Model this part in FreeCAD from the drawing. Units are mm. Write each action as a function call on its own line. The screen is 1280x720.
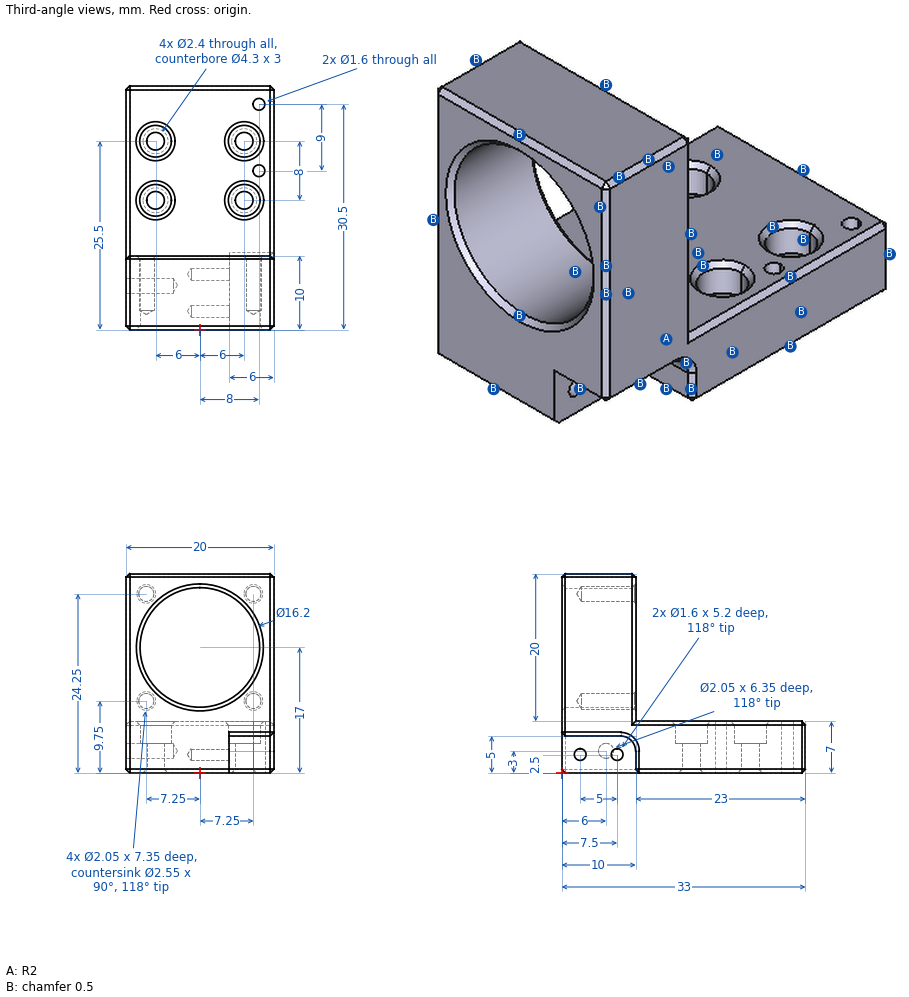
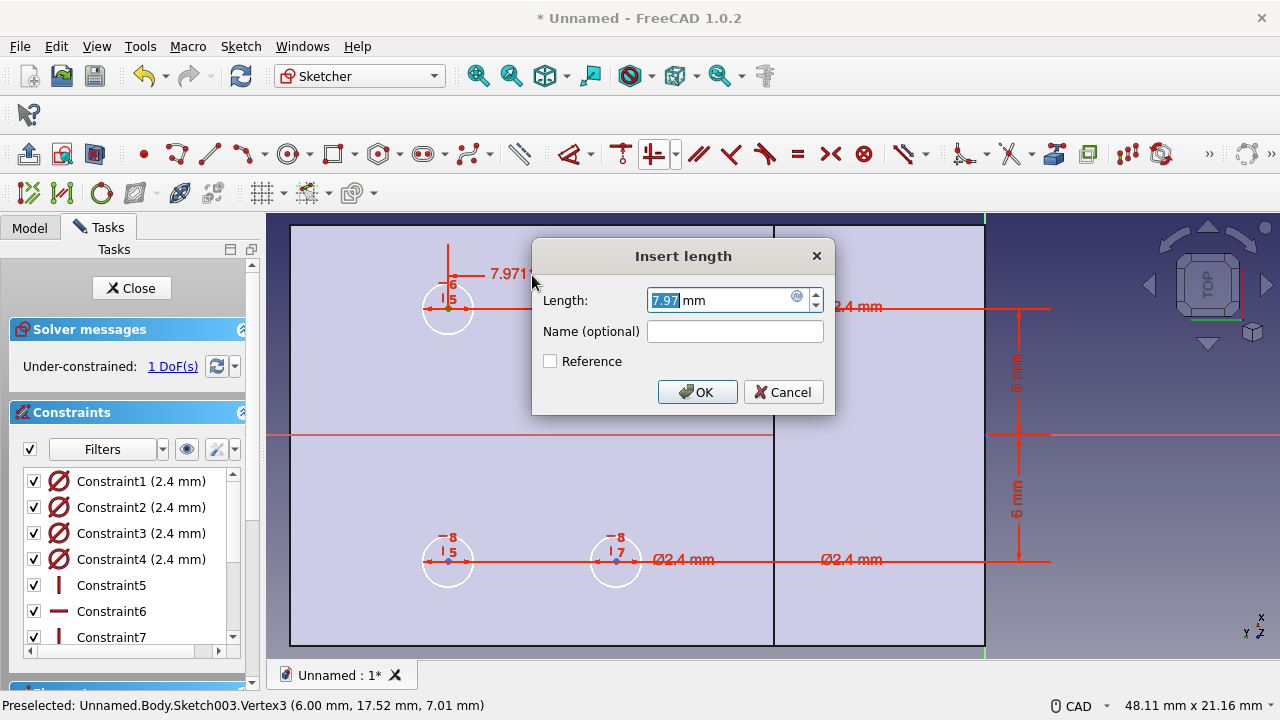
text(8)
key(Return)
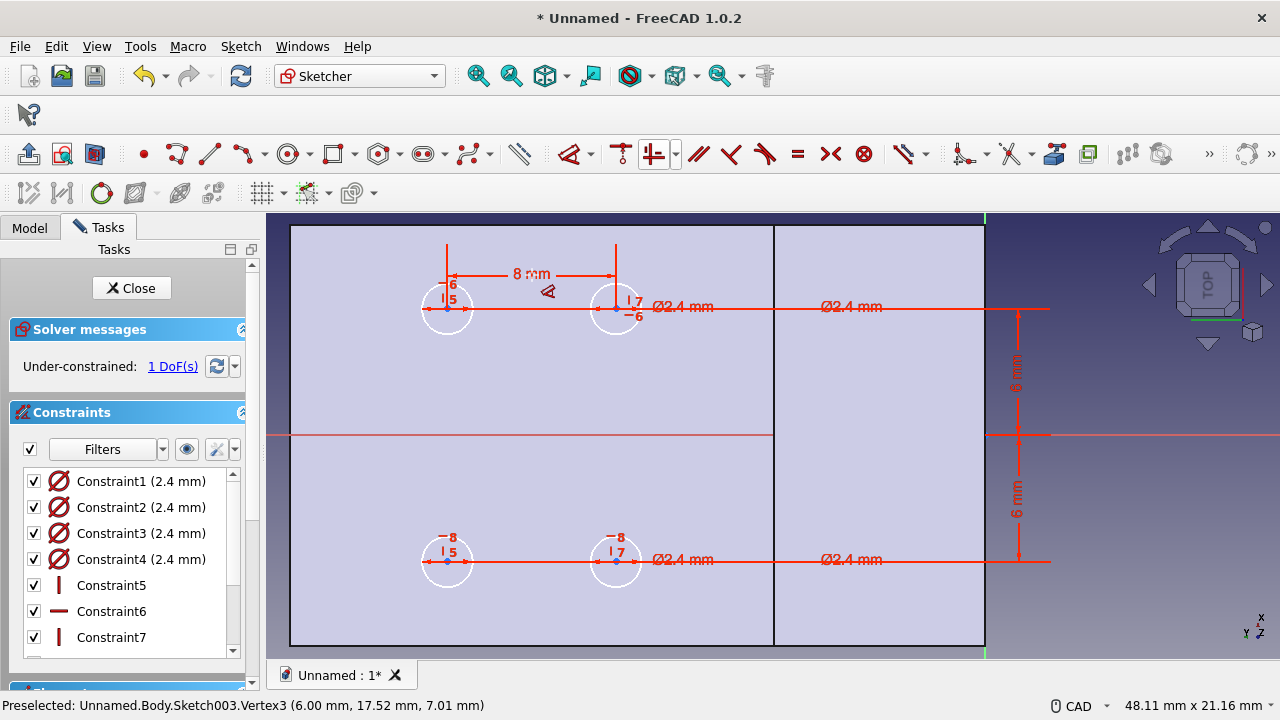
click(447, 562)
click(716, 596)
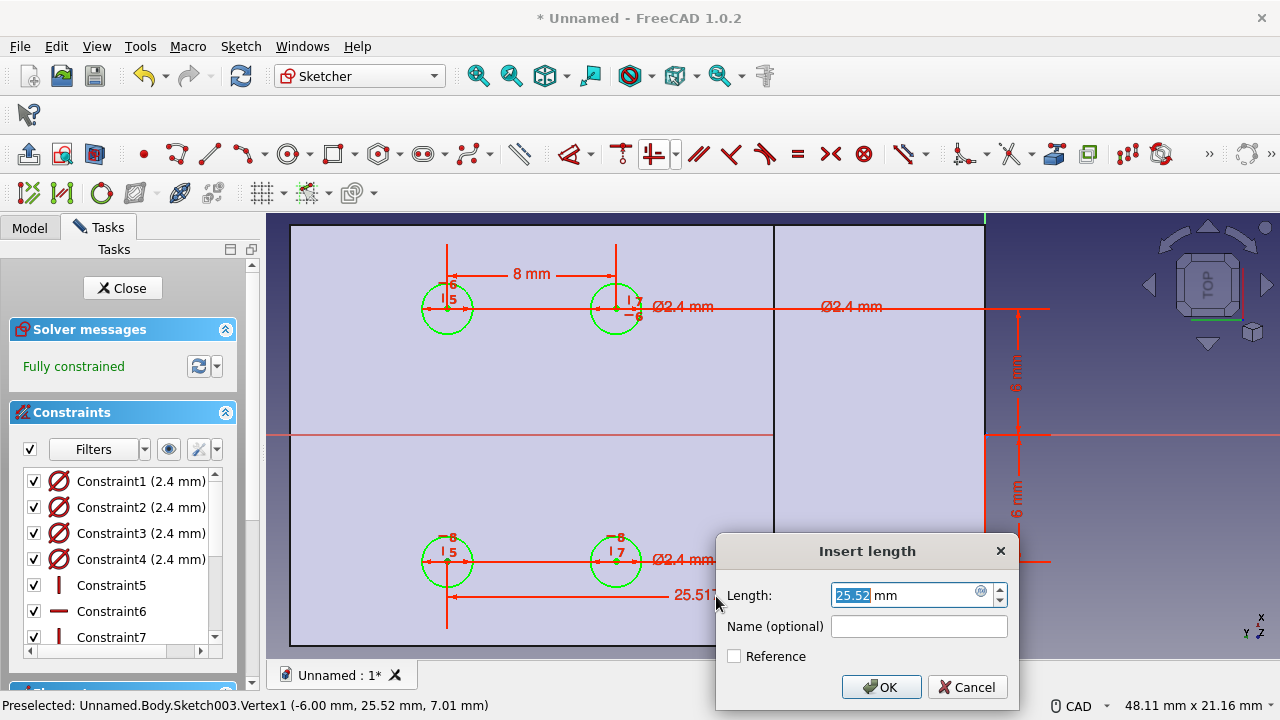
text(25.5)
key(Return)
key(Escape)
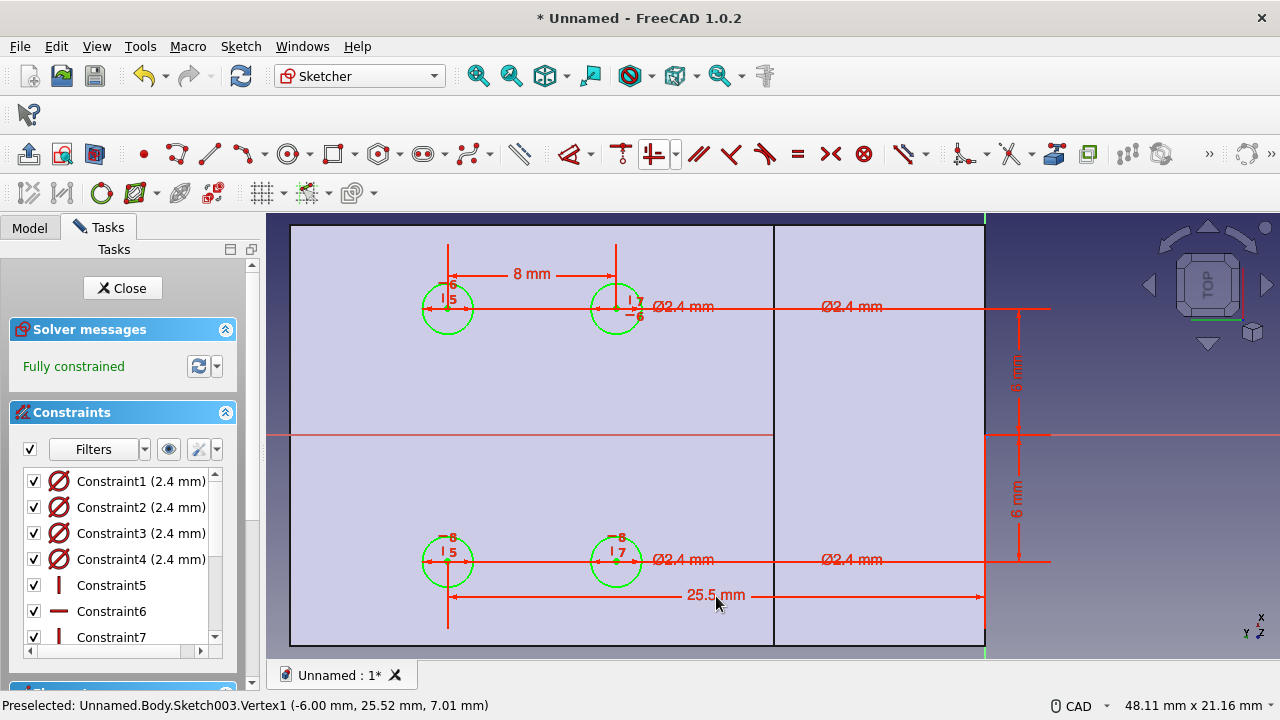
click(123, 288)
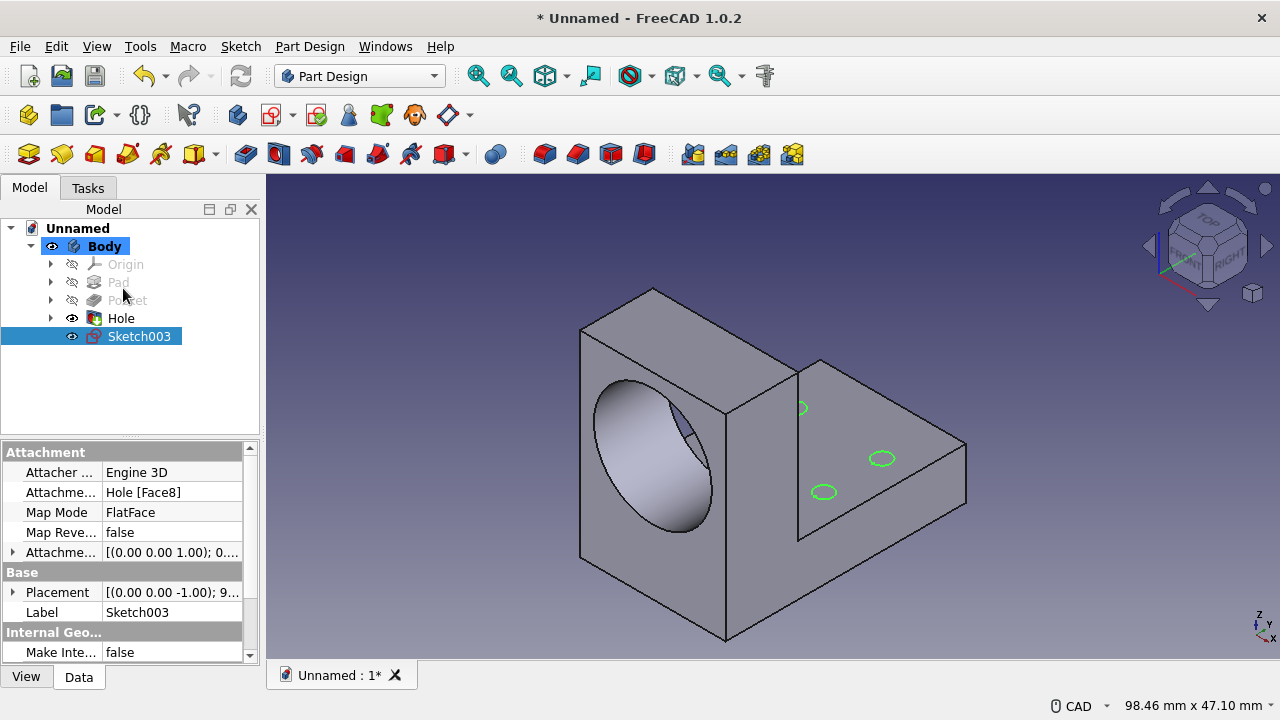
click(279, 154)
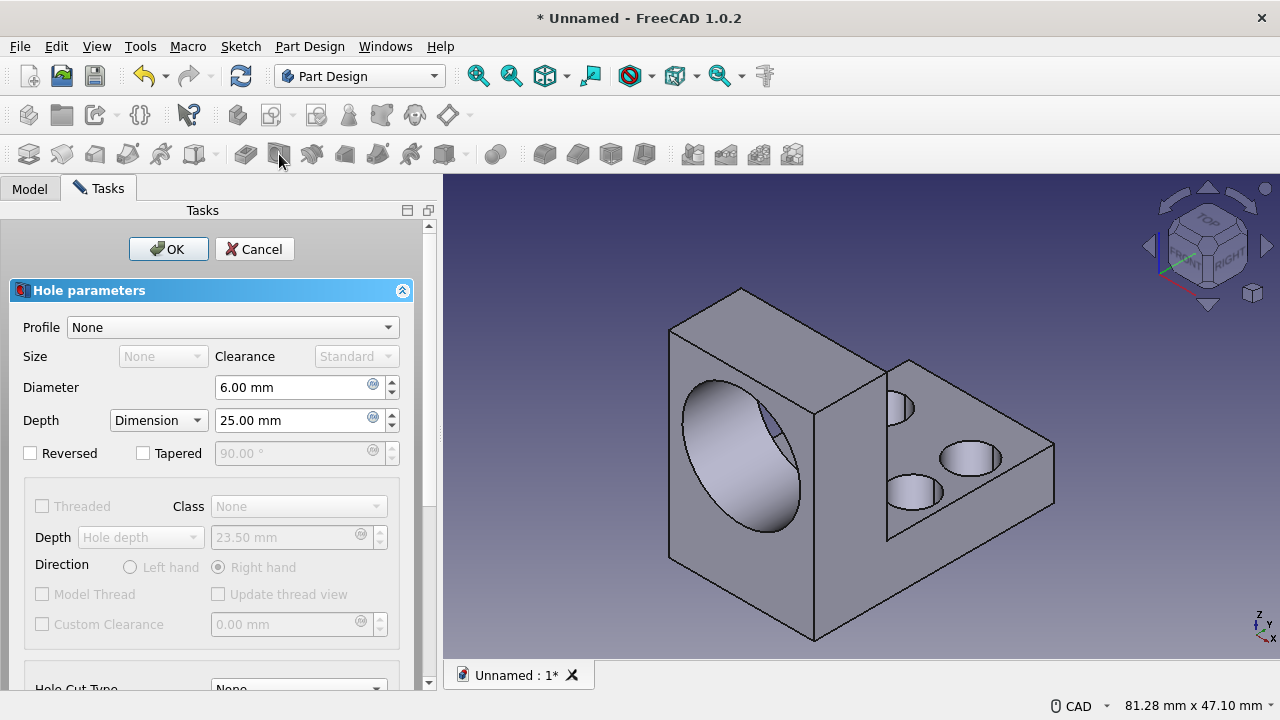
triple_click(300, 388)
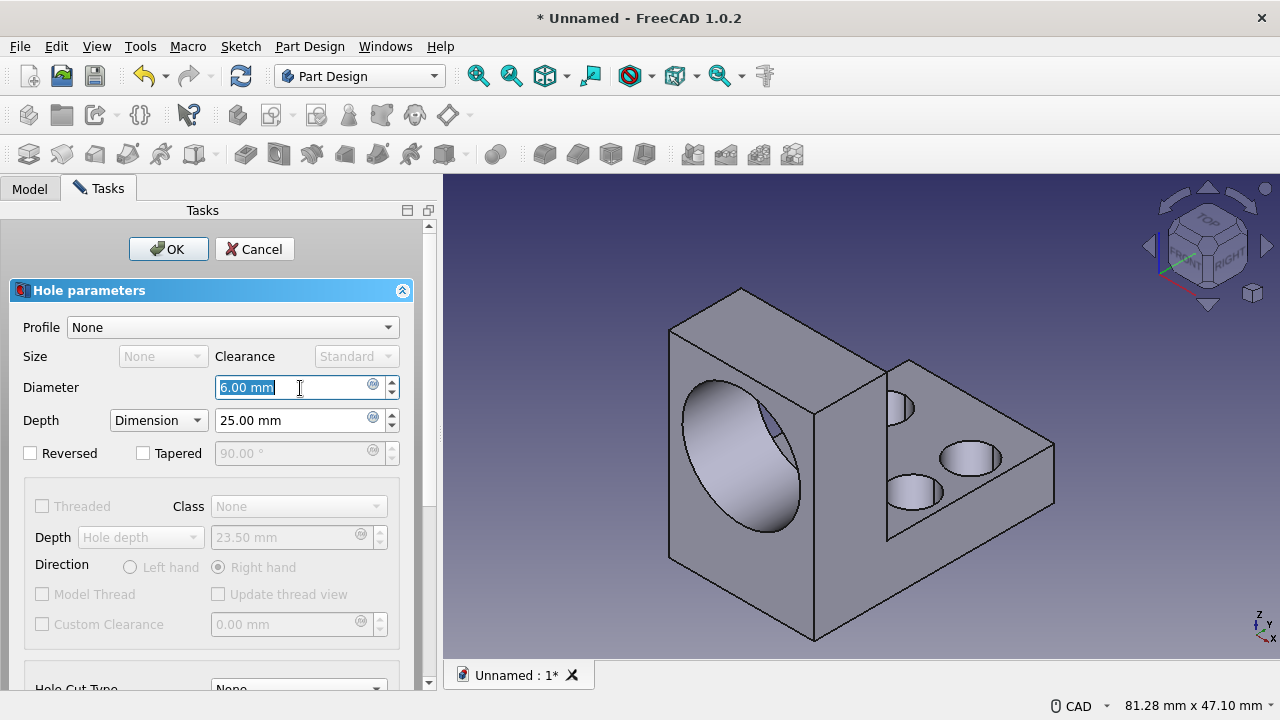
text(2.4)
key(Tab)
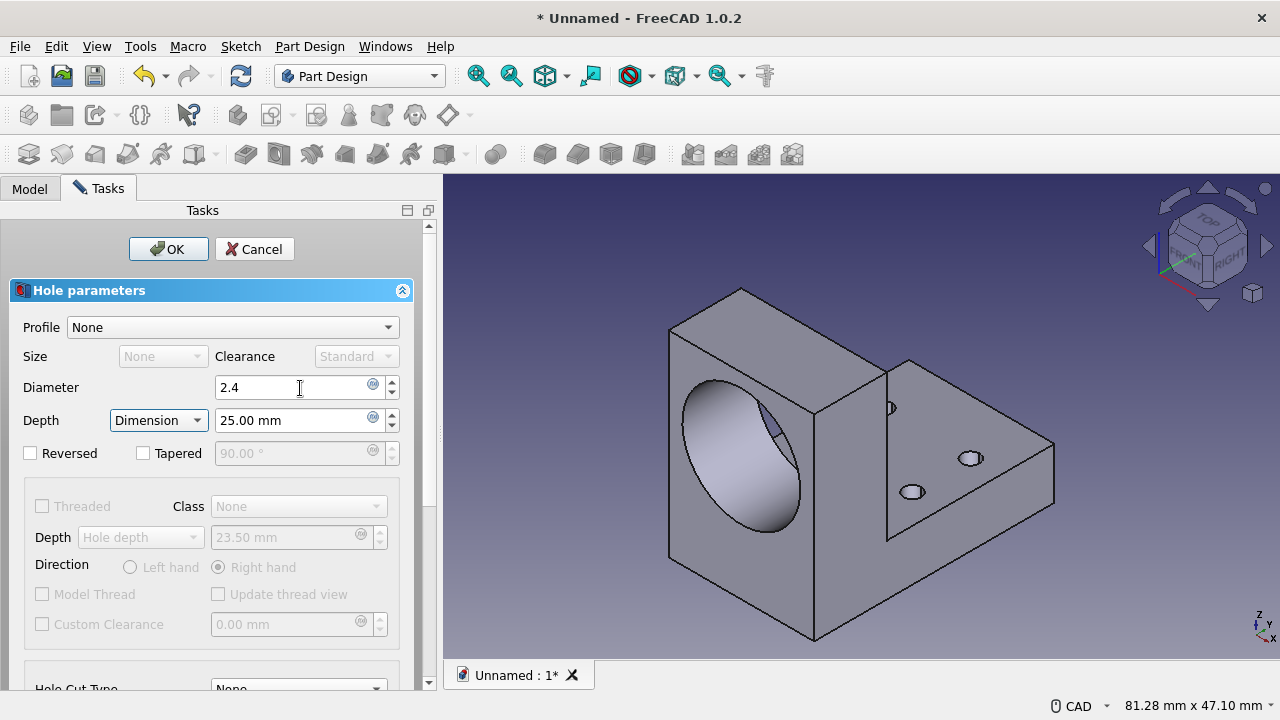
click(160, 420)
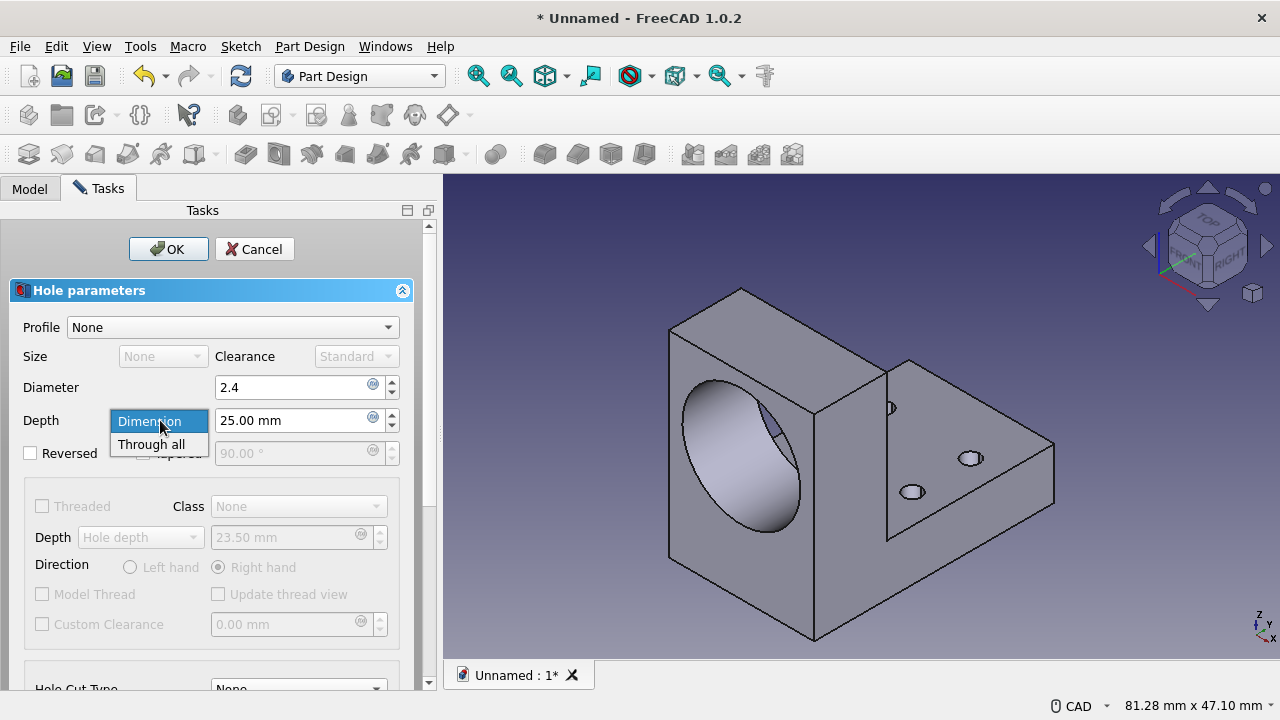
click(158, 444)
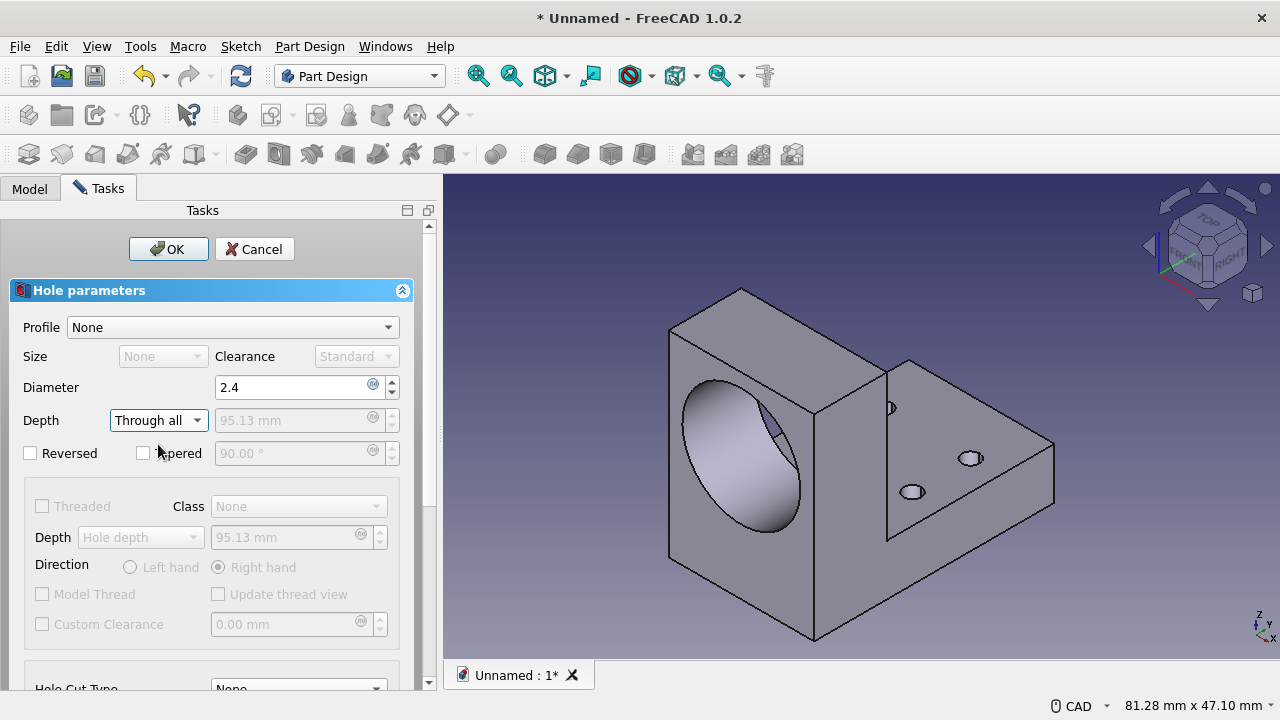
scroll(429, 455, down, 2)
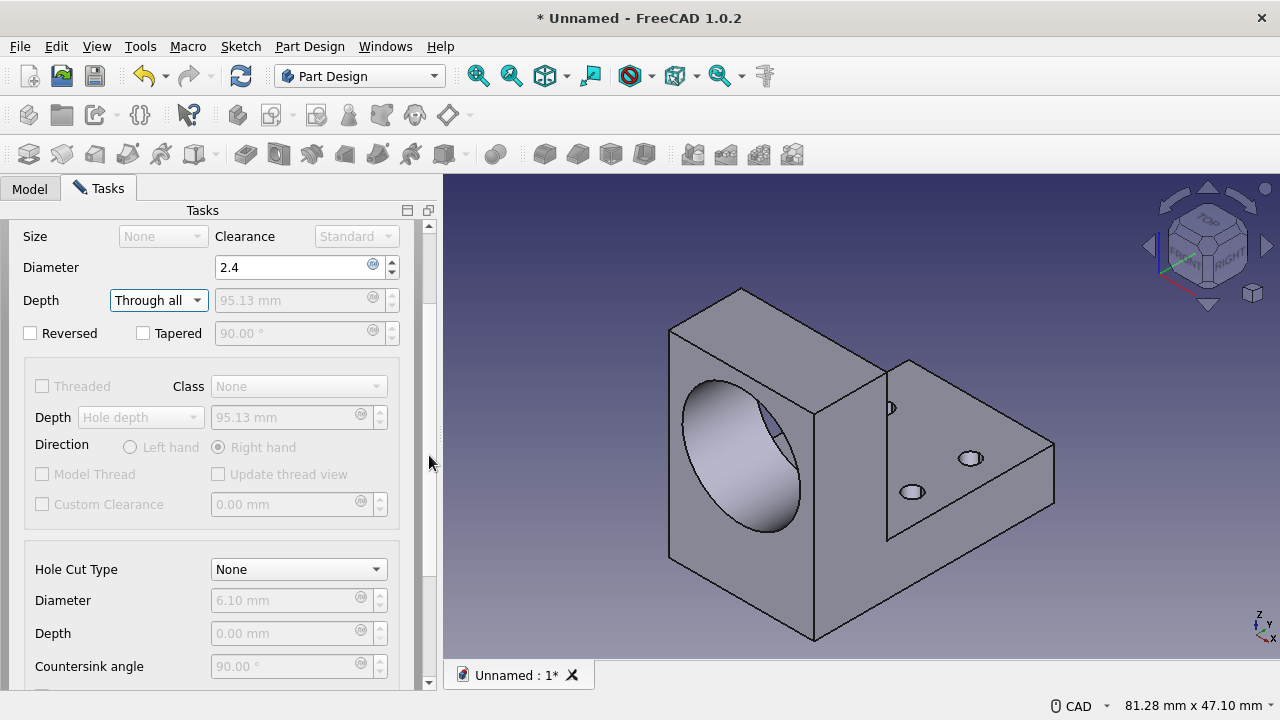
click(300, 570)